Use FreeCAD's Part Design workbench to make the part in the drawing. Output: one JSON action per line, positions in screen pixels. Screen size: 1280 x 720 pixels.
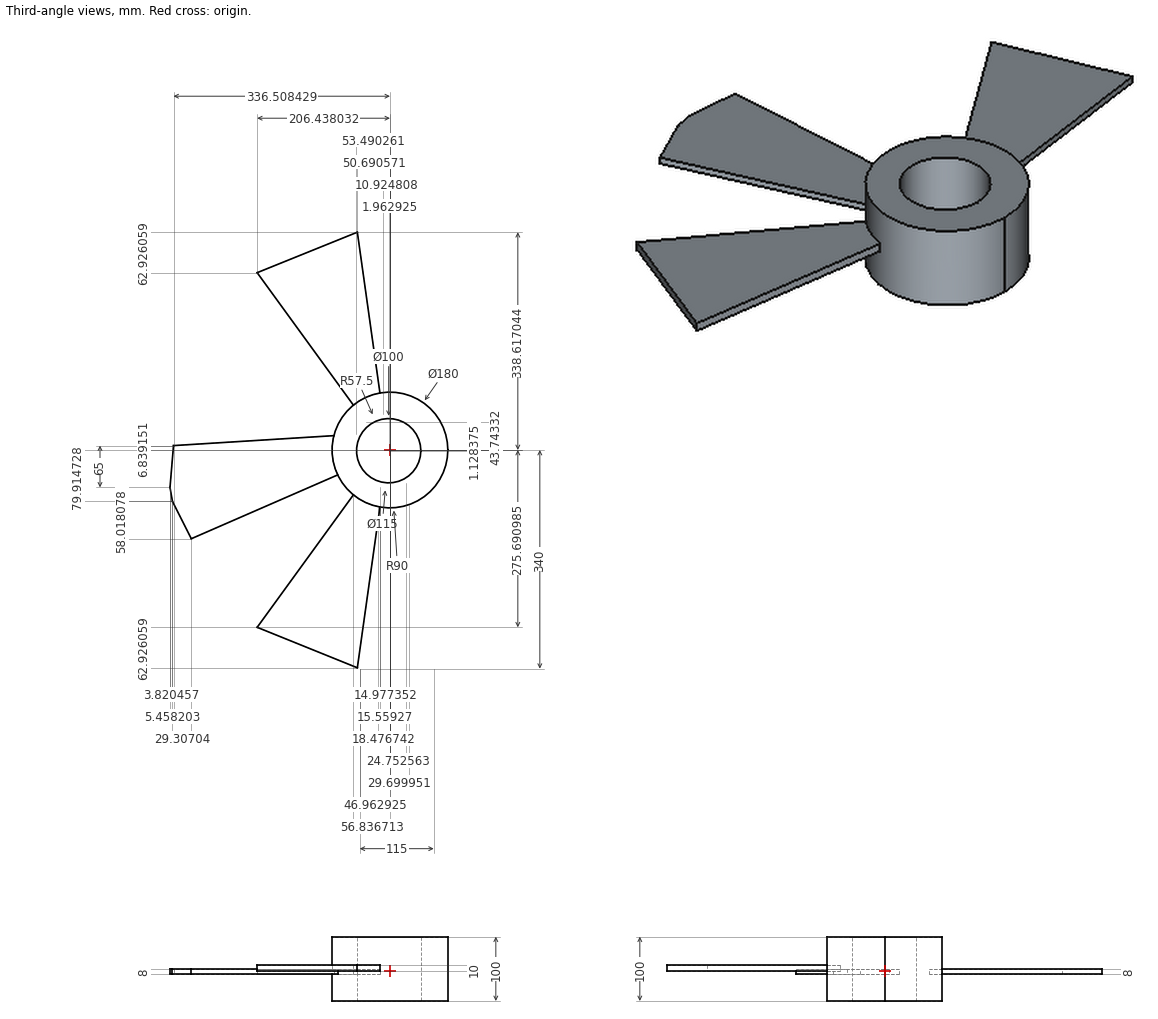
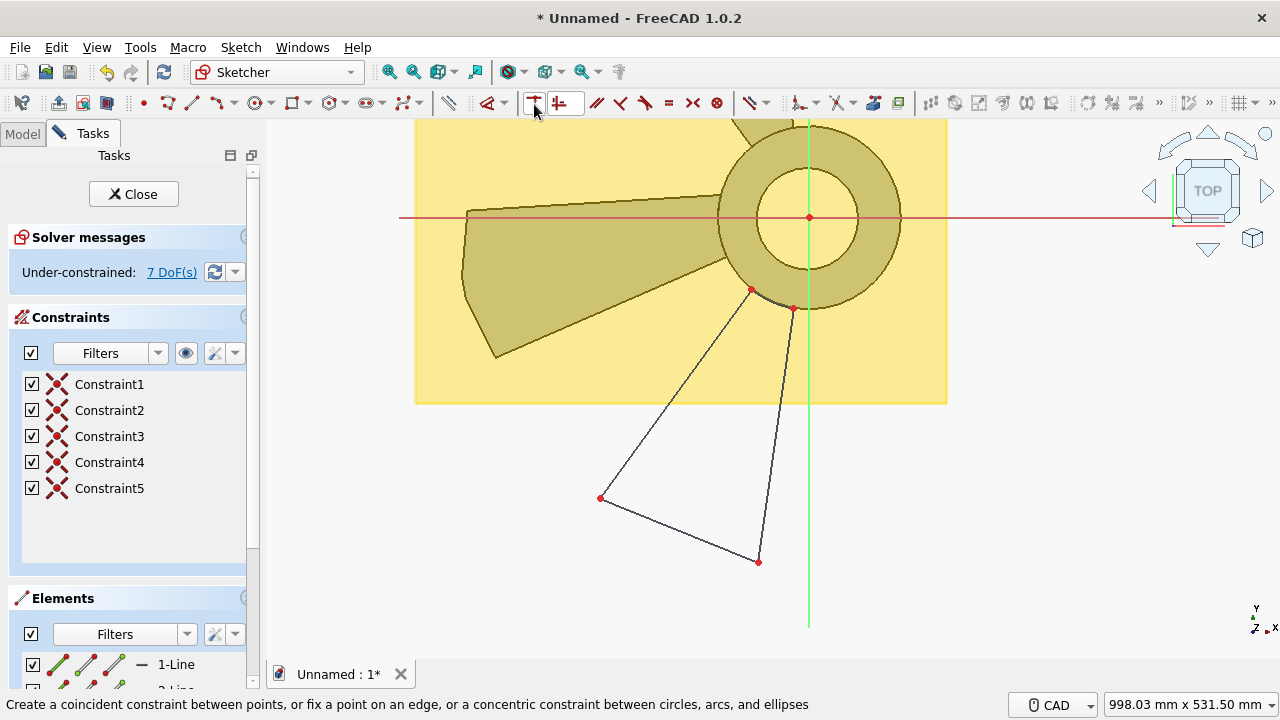
{"action": "left_click", "coordinate": [488, 104]}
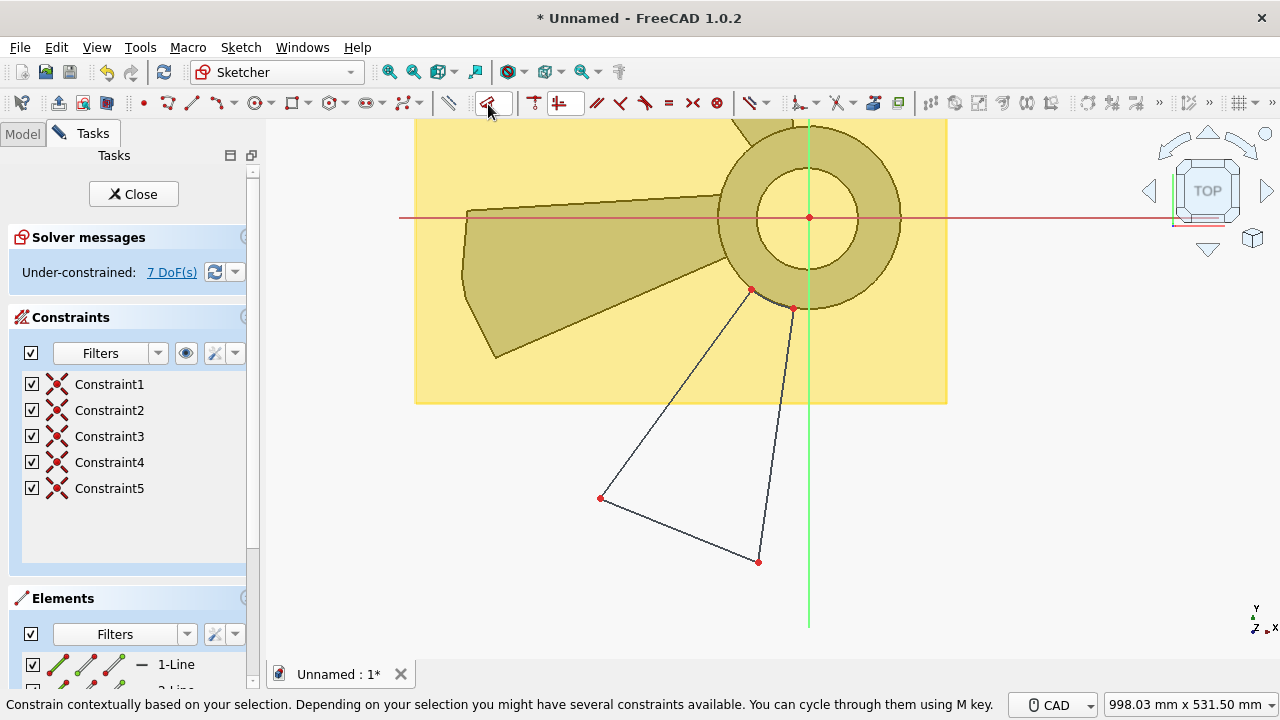
{"action": "left_click", "coordinate": [764, 298]}
{"action": "left_click", "coordinate": [748, 326]}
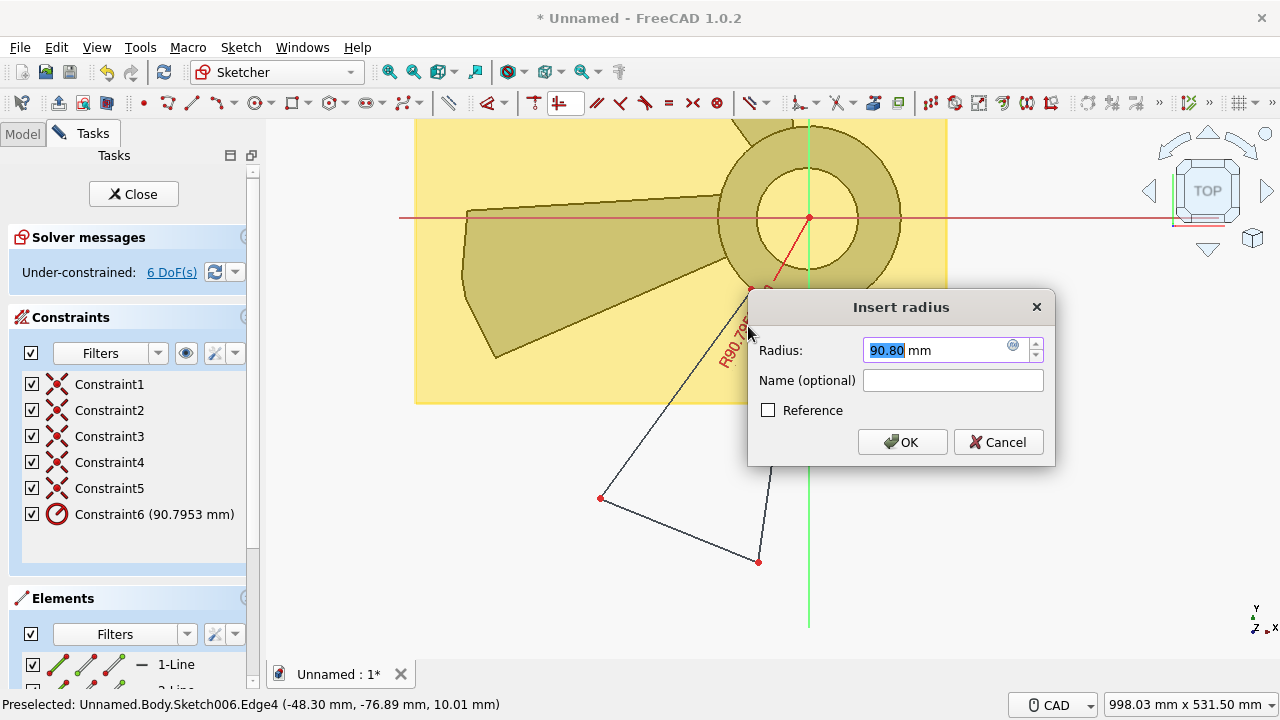
{"action": "type", "text": "90"}
{"action": "key", "text": "Return"}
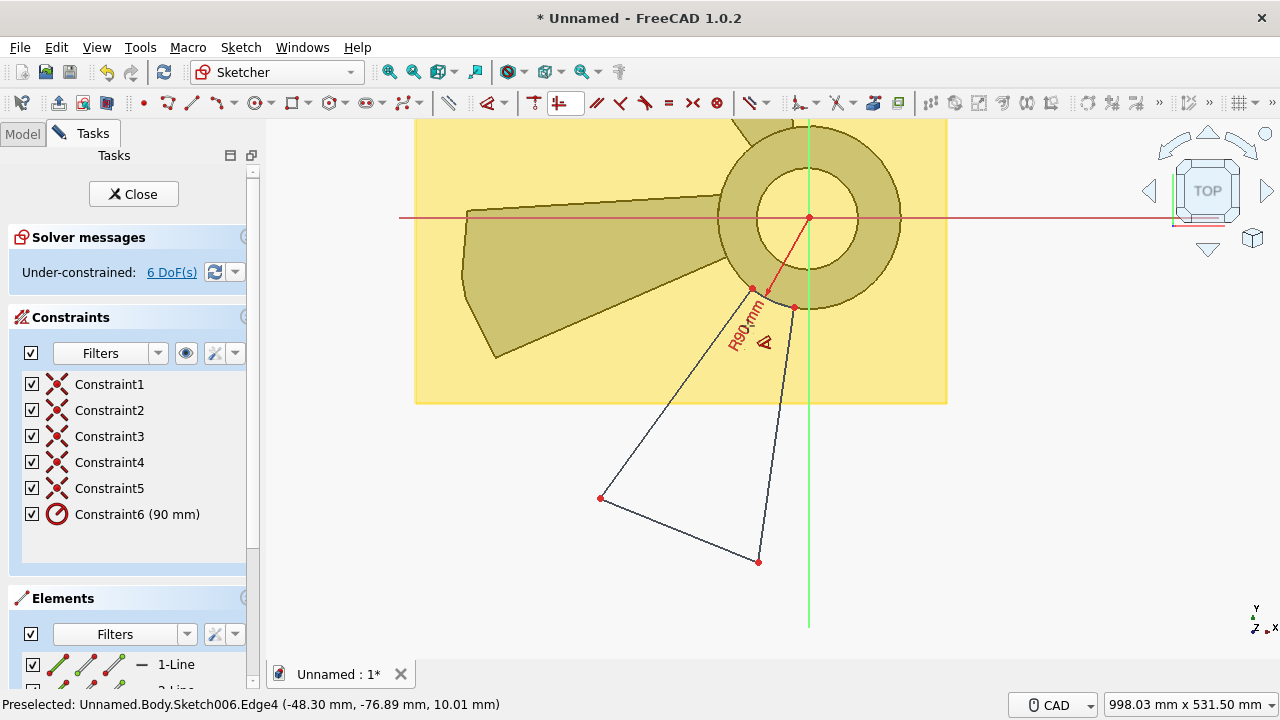
{"action": "scroll", "coordinate": [794, 308], "scroll_direction": "up", "scroll_amount": 5}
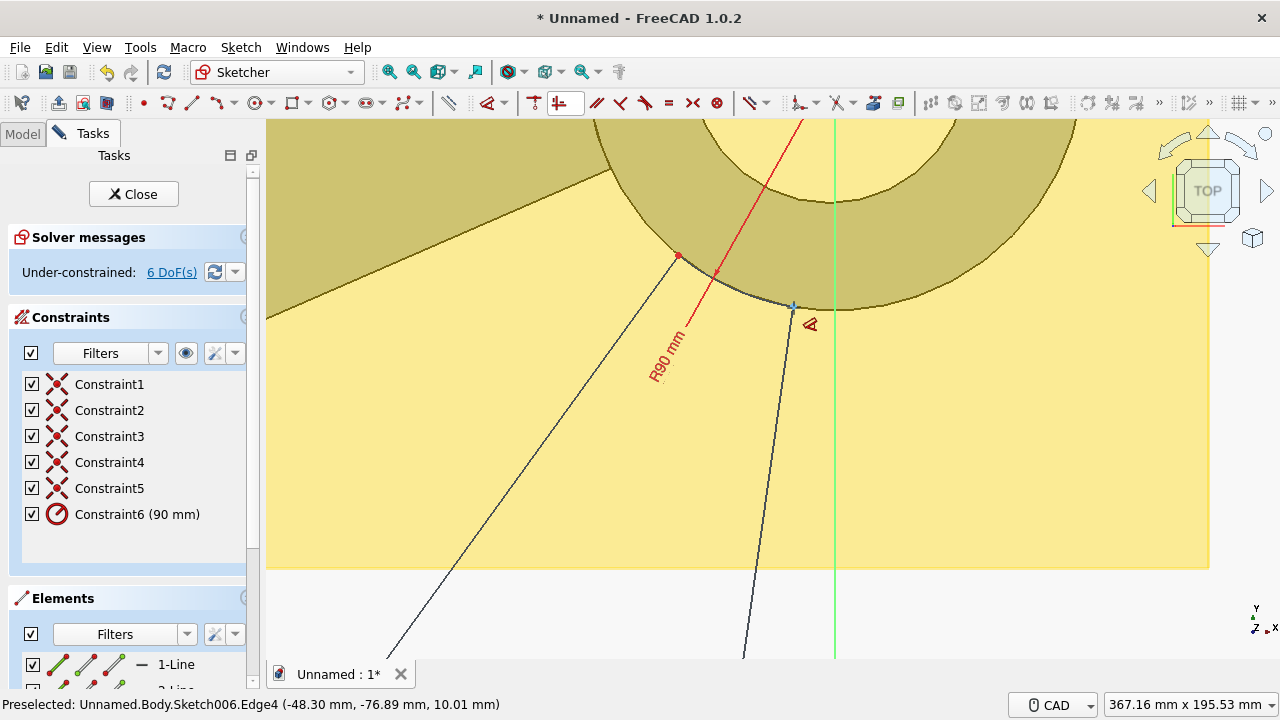
{"action": "left_click", "coordinate": [793, 307]}
{"action": "left_click", "coordinate": [814, 341]}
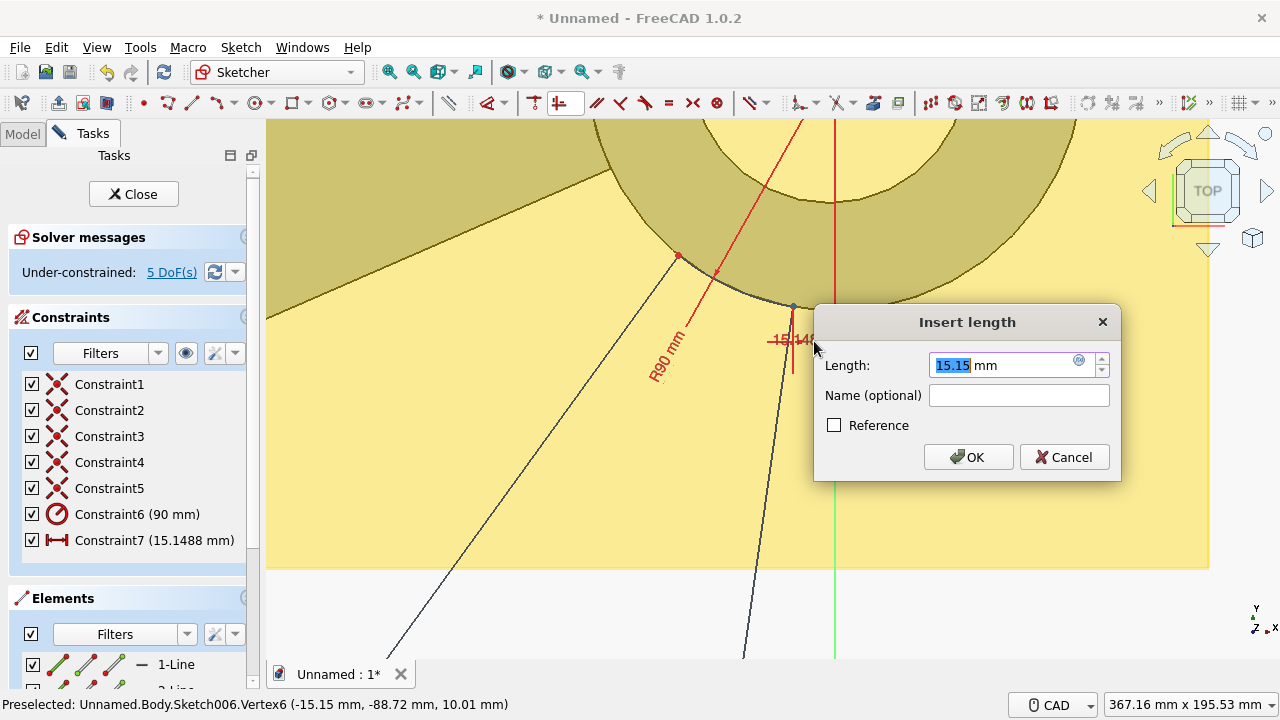
{"action": "type", "text": "15.55927"}
{"action": "key", "text": "Return"}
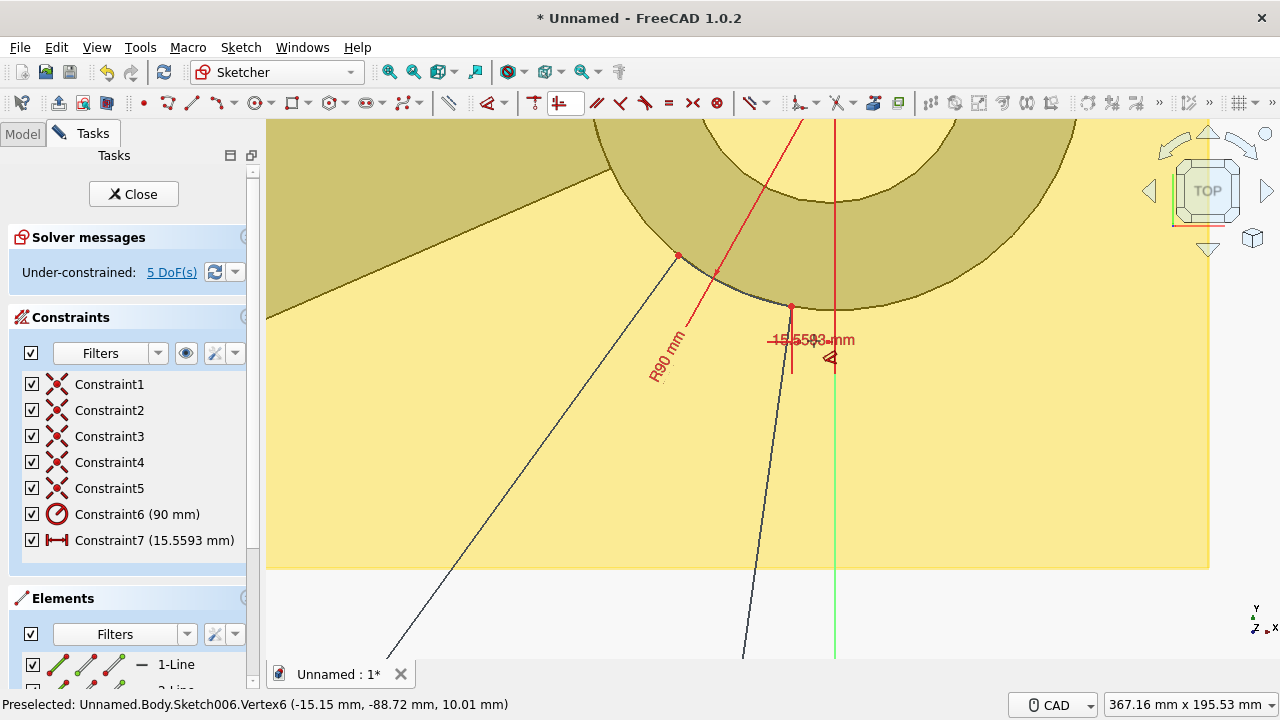
{"action": "left_click", "coordinate": [679, 255]}
{"action": "left_click", "coordinate": [793, 289]}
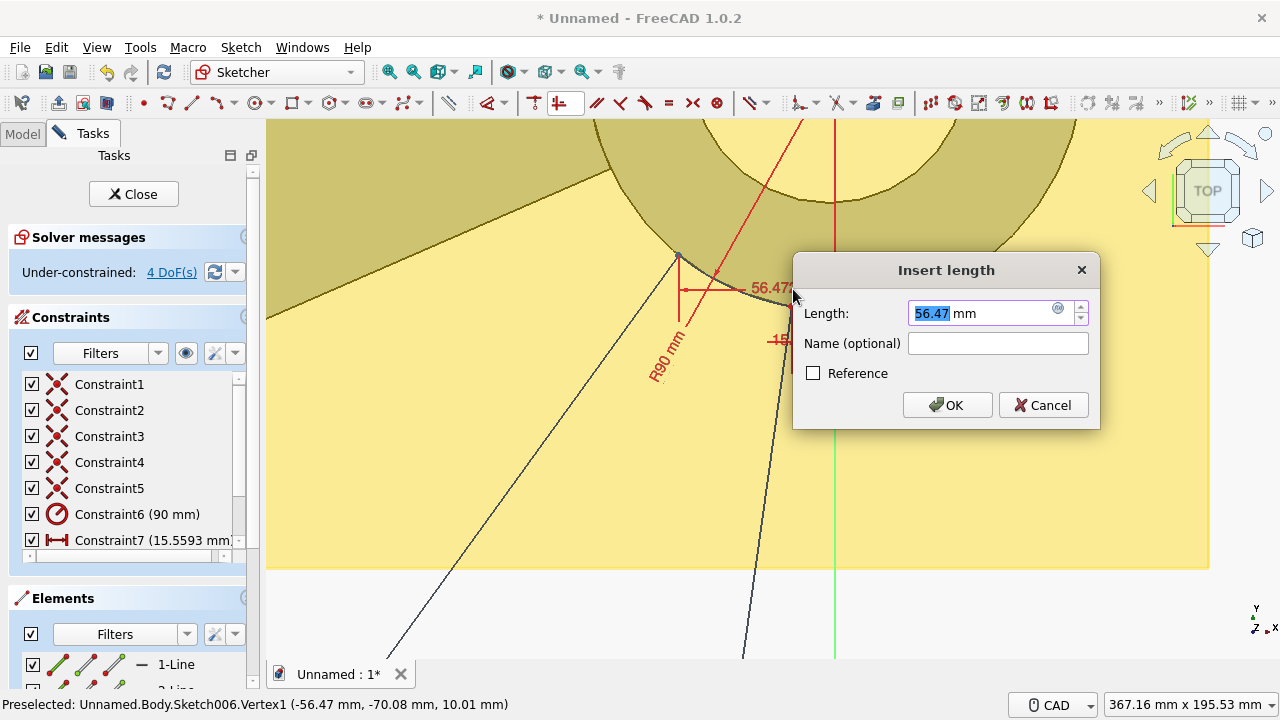
{"action": "type", "text": "56.836713"}
{"action": "key", "text": "Return"}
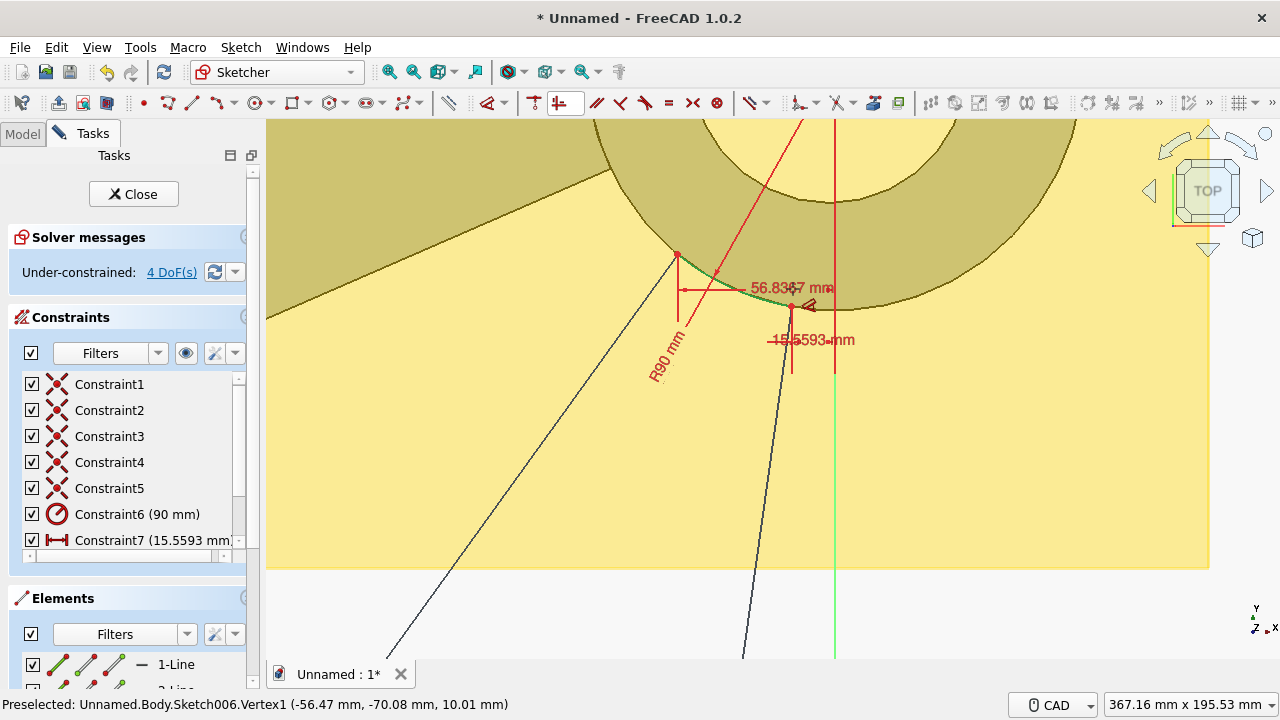
{"action": "scroll", "coordinate": [794, 307], "scroll_direction": "down", "scroll_amount": 5}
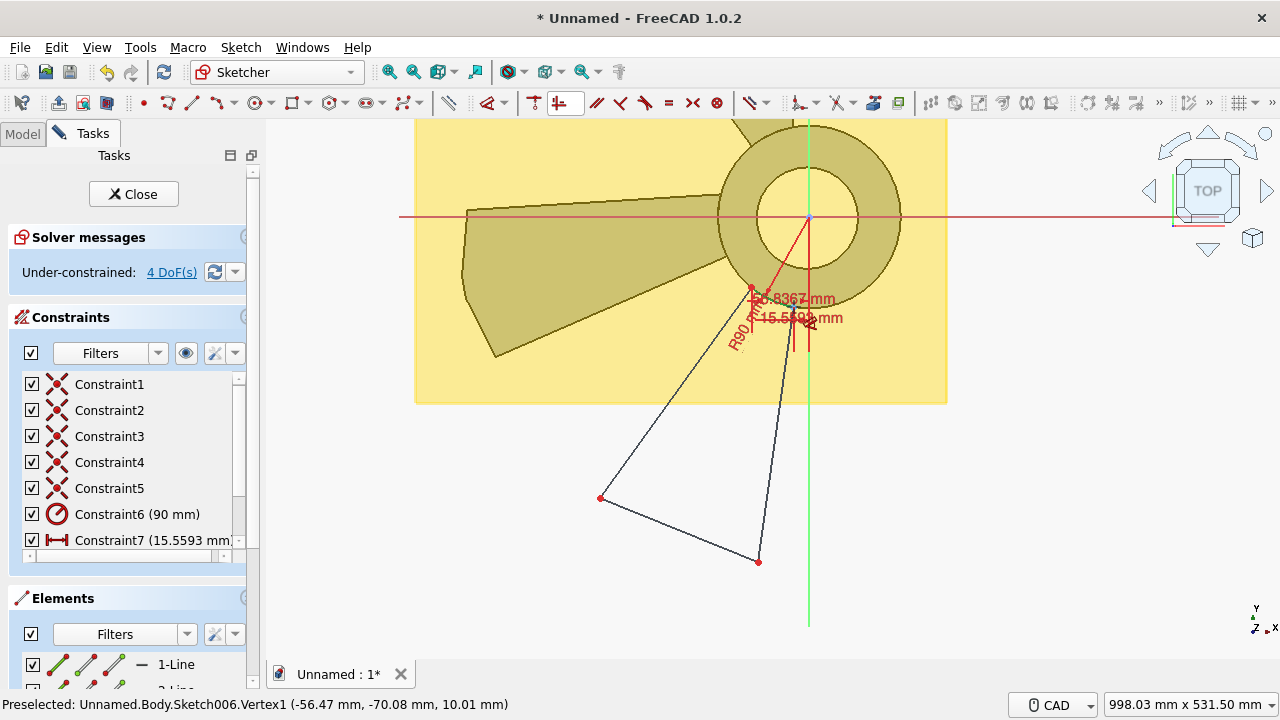
{"action": "left_click", "coordinate": [758, 562]}
{"action": "left_click", "coordinate": [784, 596]}